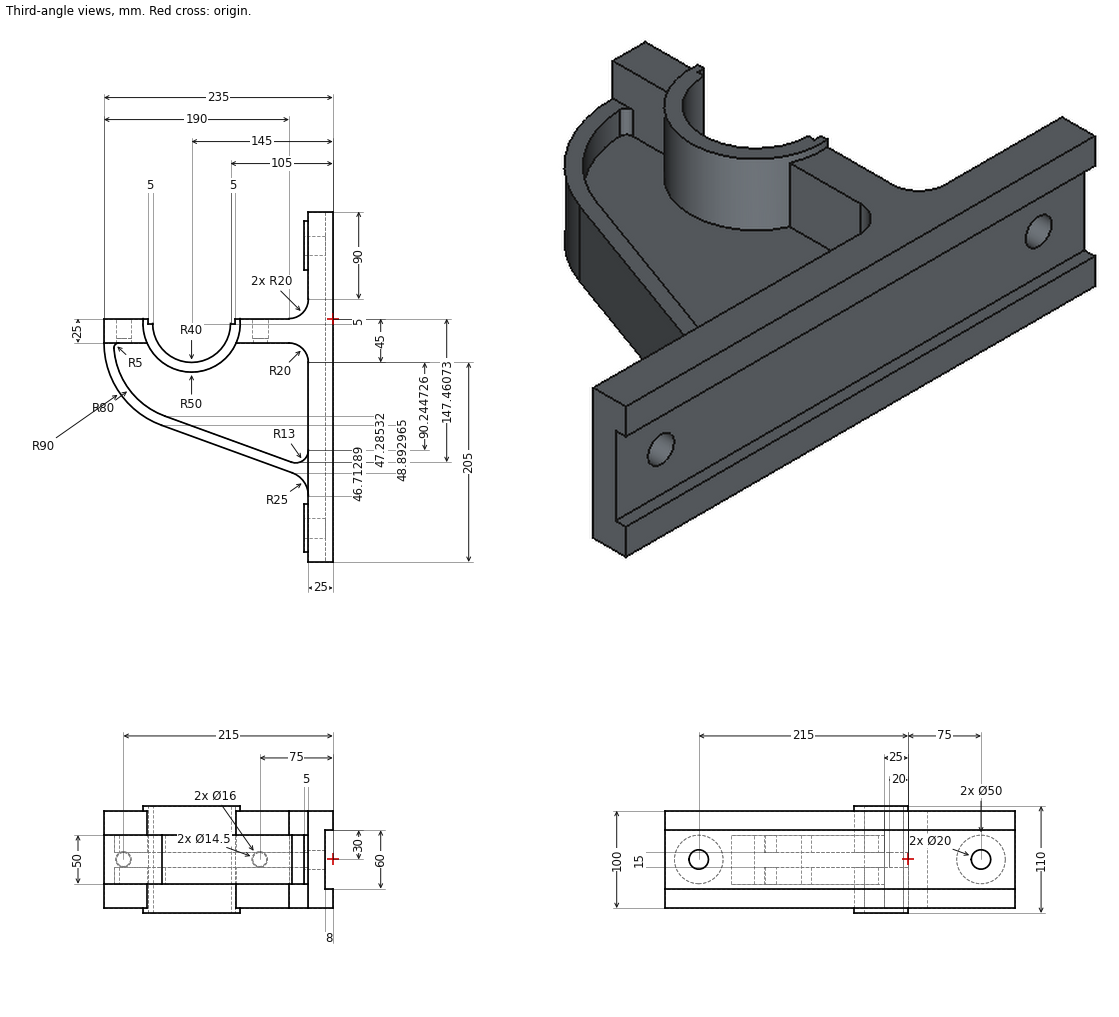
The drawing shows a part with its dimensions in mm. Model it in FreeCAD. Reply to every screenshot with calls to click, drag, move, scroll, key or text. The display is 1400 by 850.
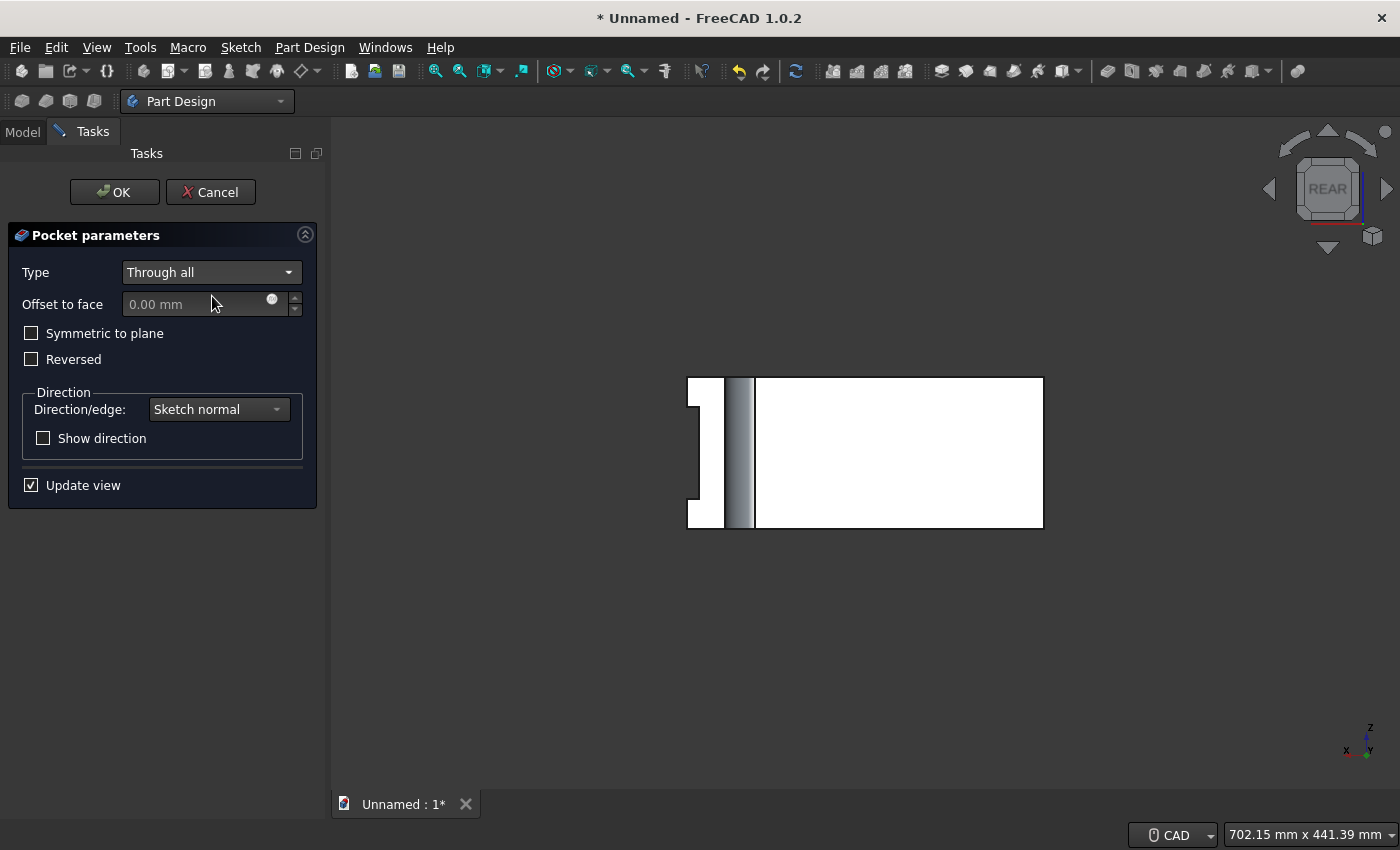
click(115, 192)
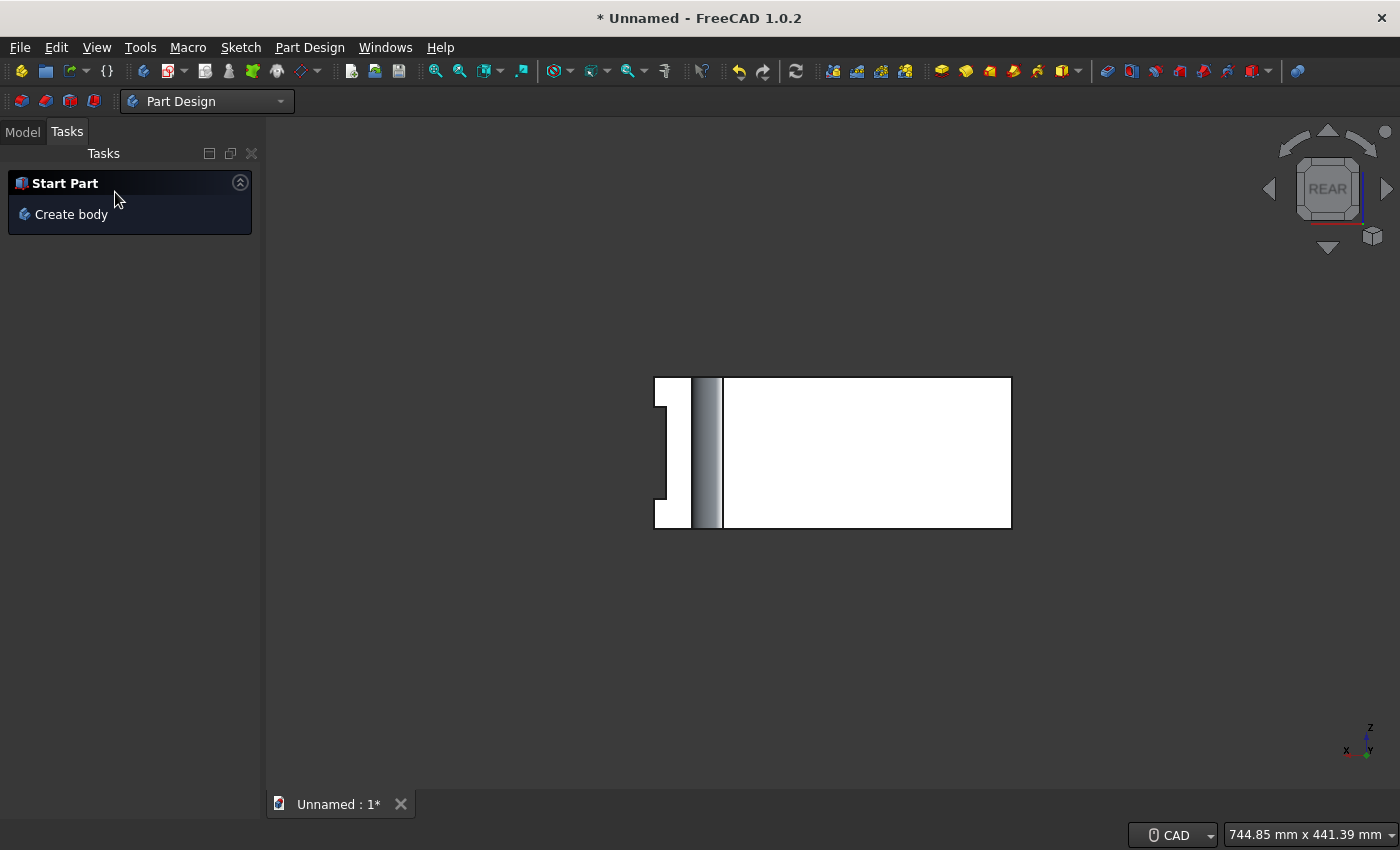
click(436, 72)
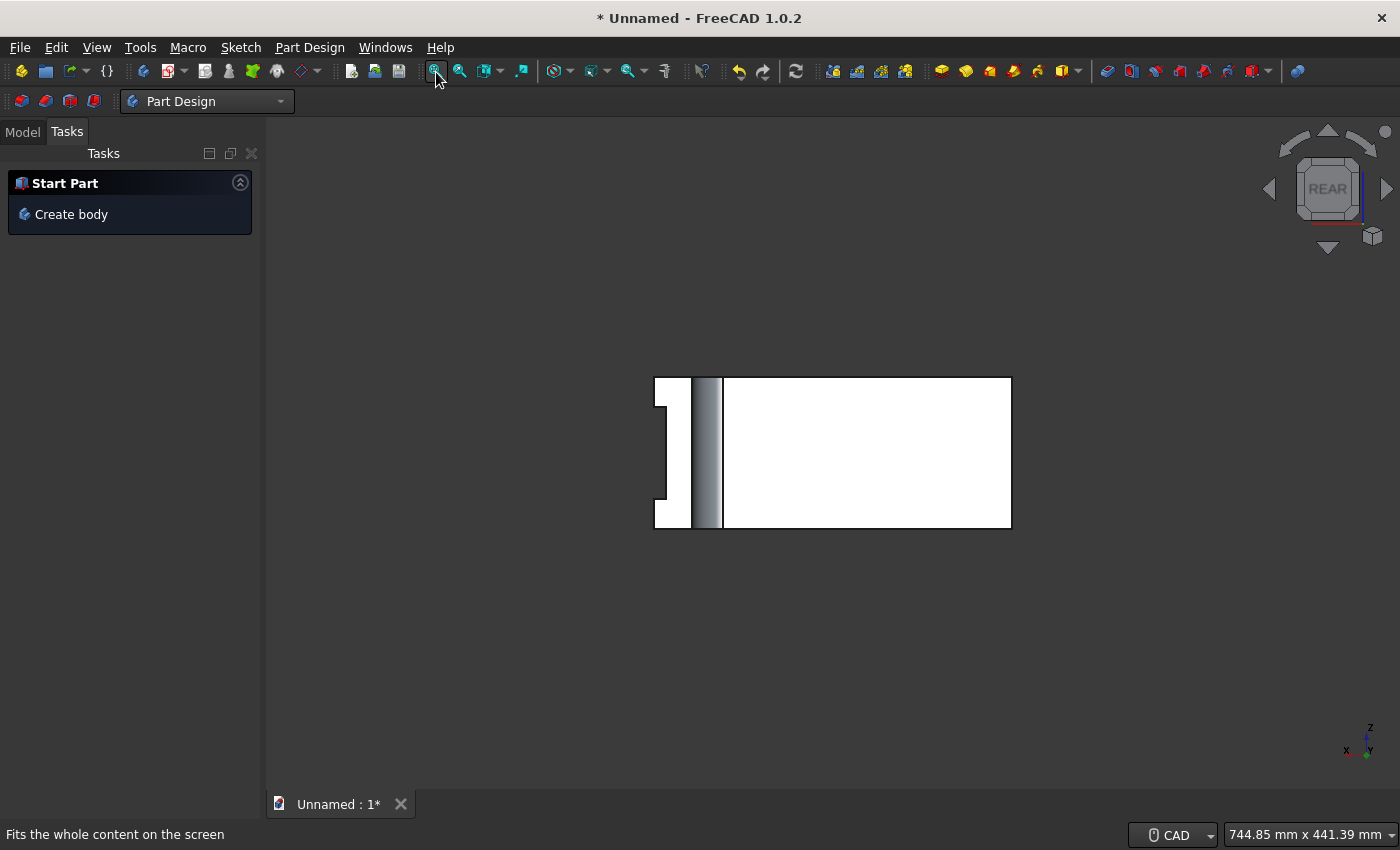
key(6)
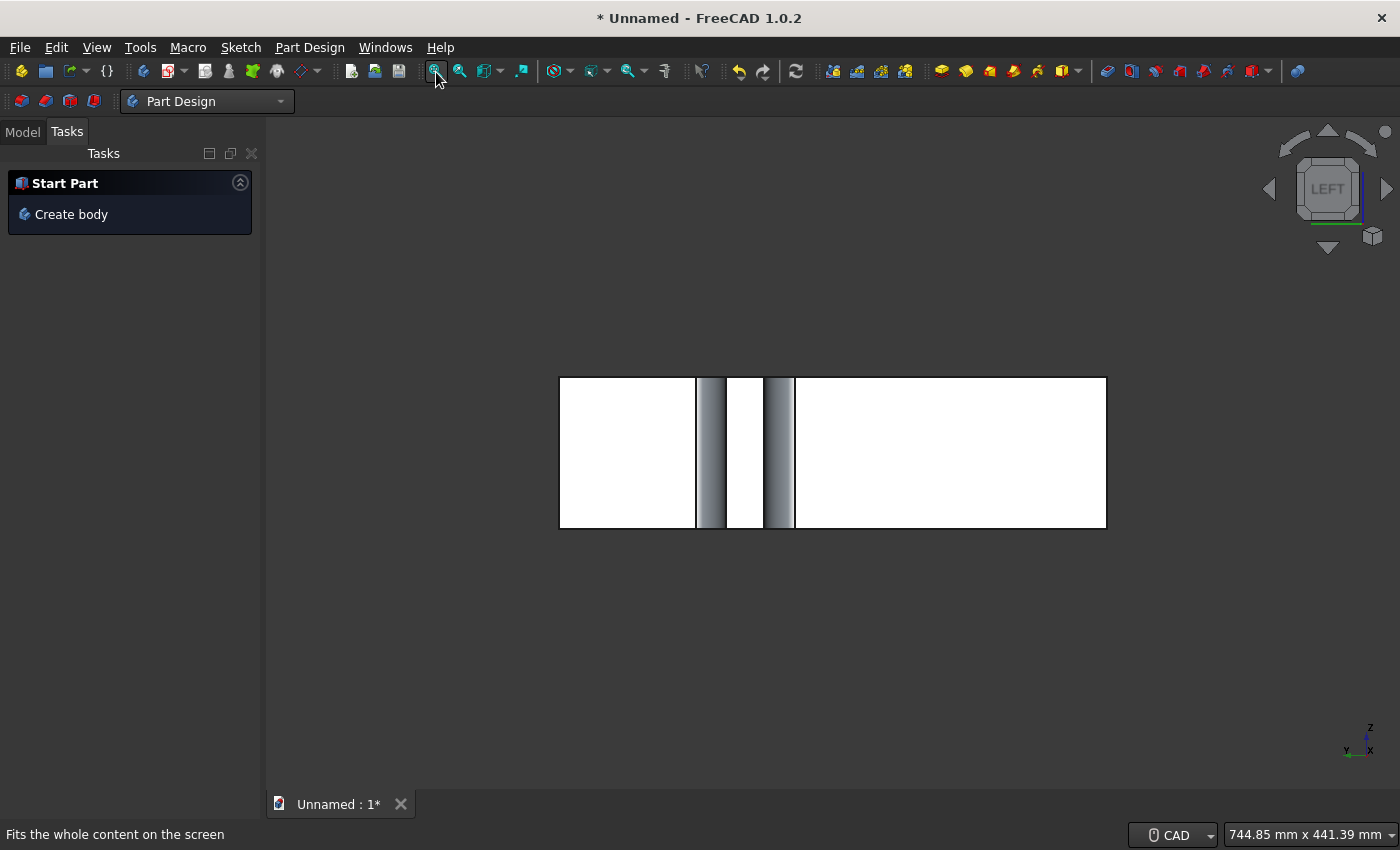
click(906, 452)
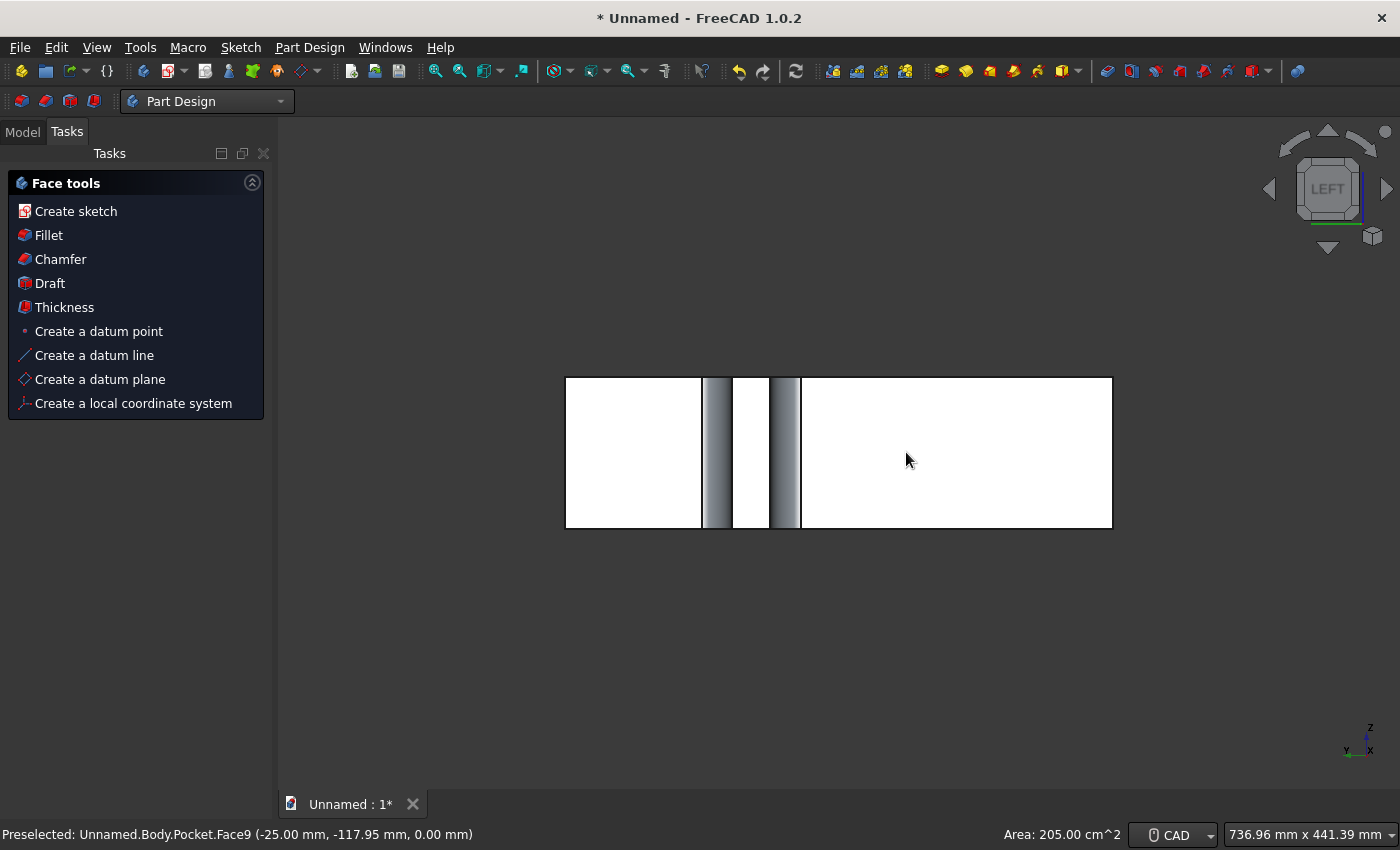
click(168, 72)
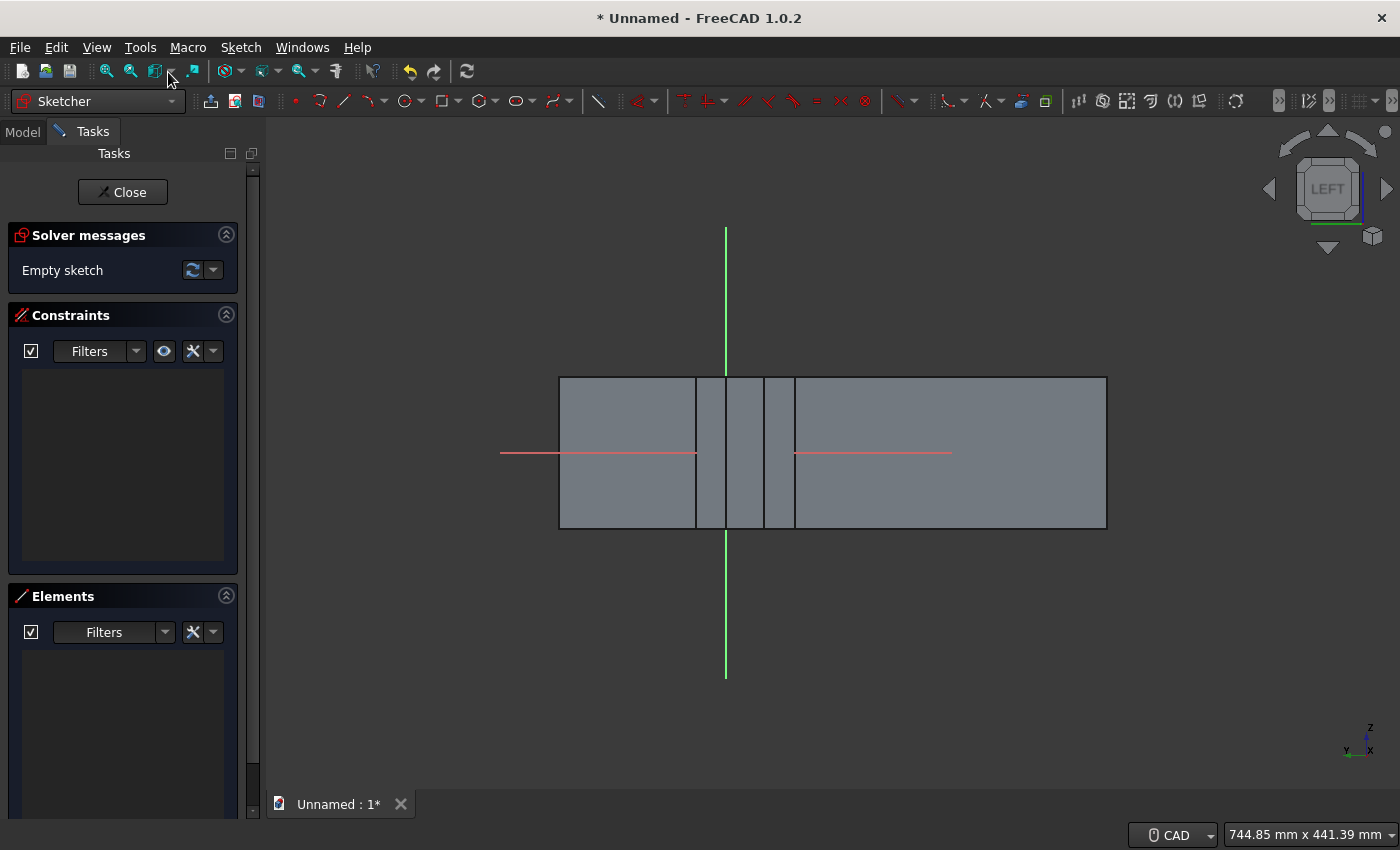
click(260, 102)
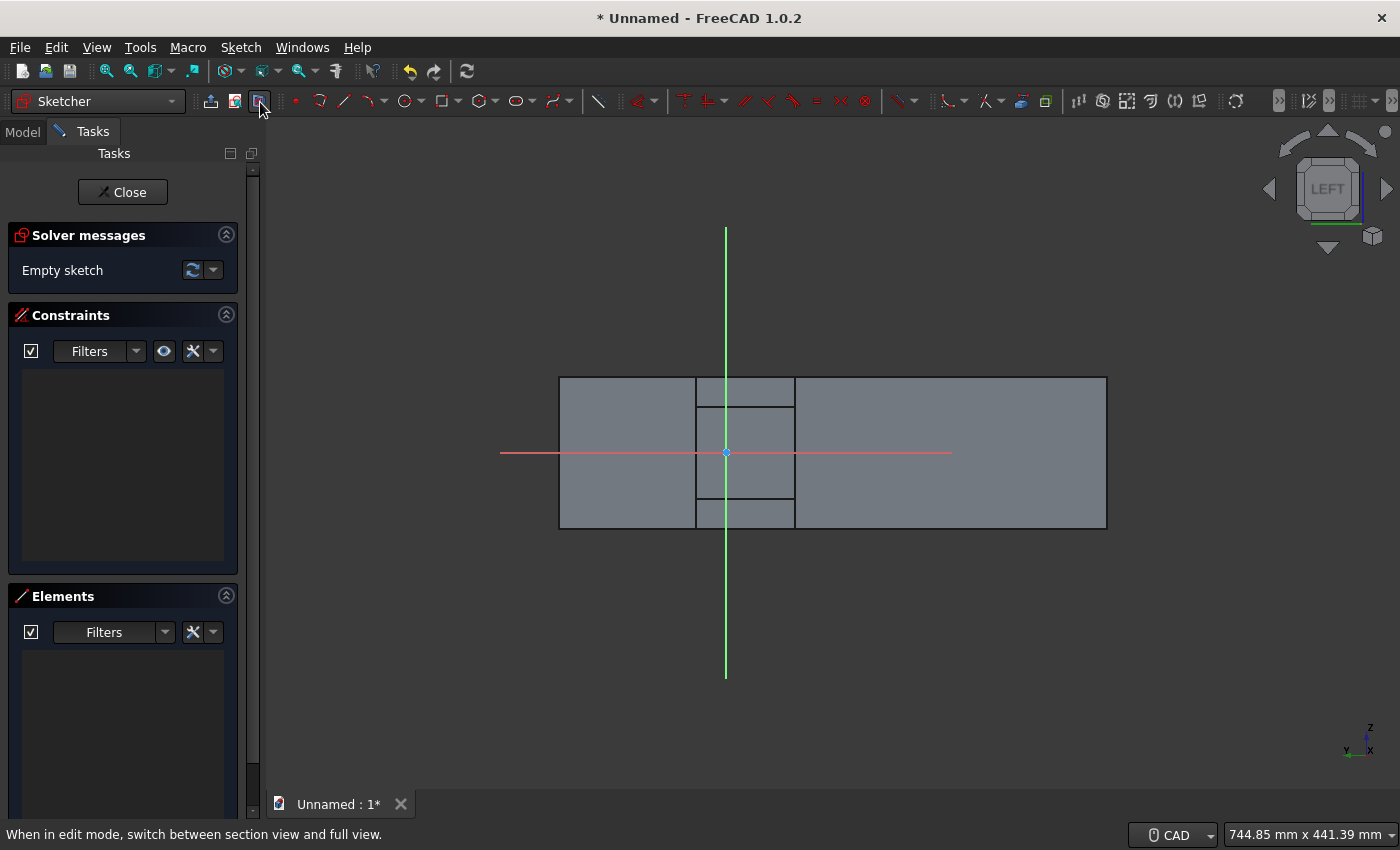
click(406, 102)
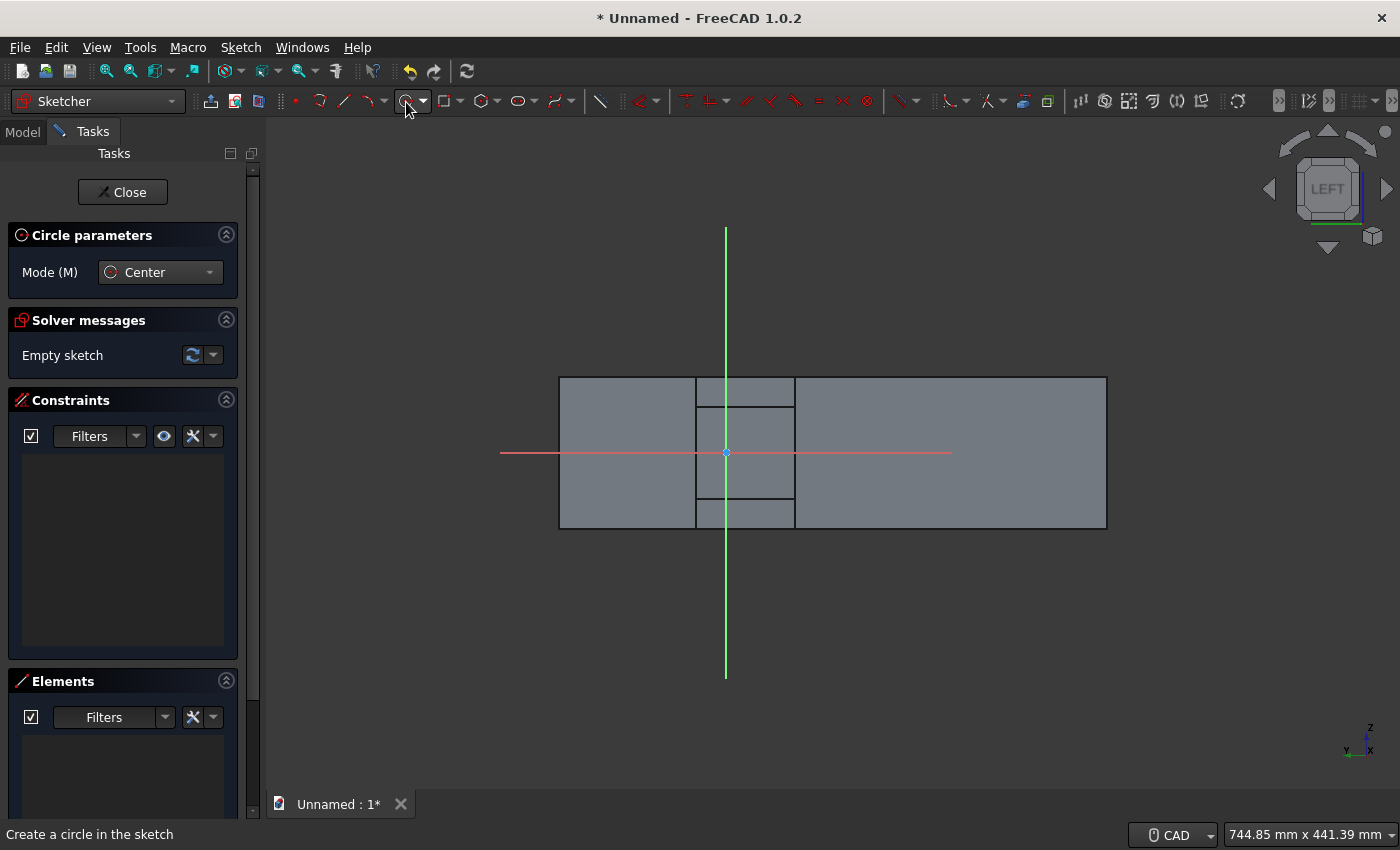
click(612, 453)
move(639, 426)